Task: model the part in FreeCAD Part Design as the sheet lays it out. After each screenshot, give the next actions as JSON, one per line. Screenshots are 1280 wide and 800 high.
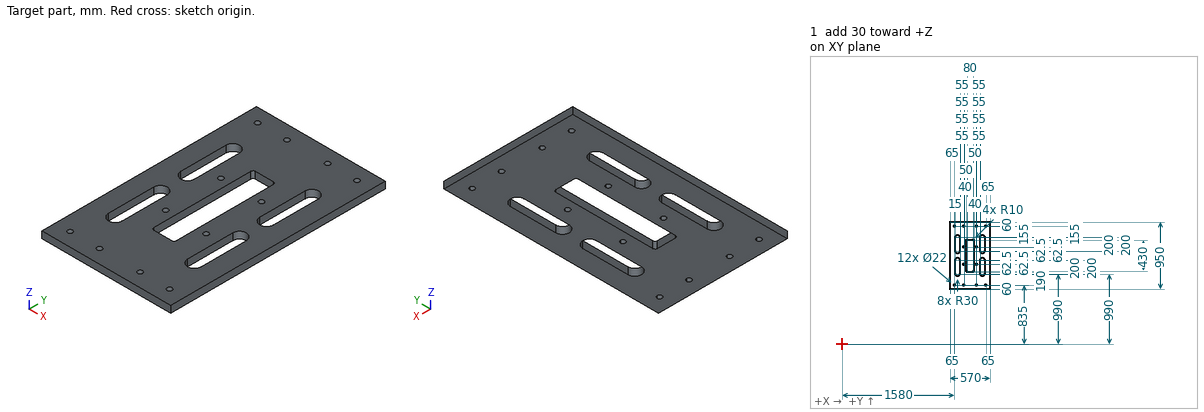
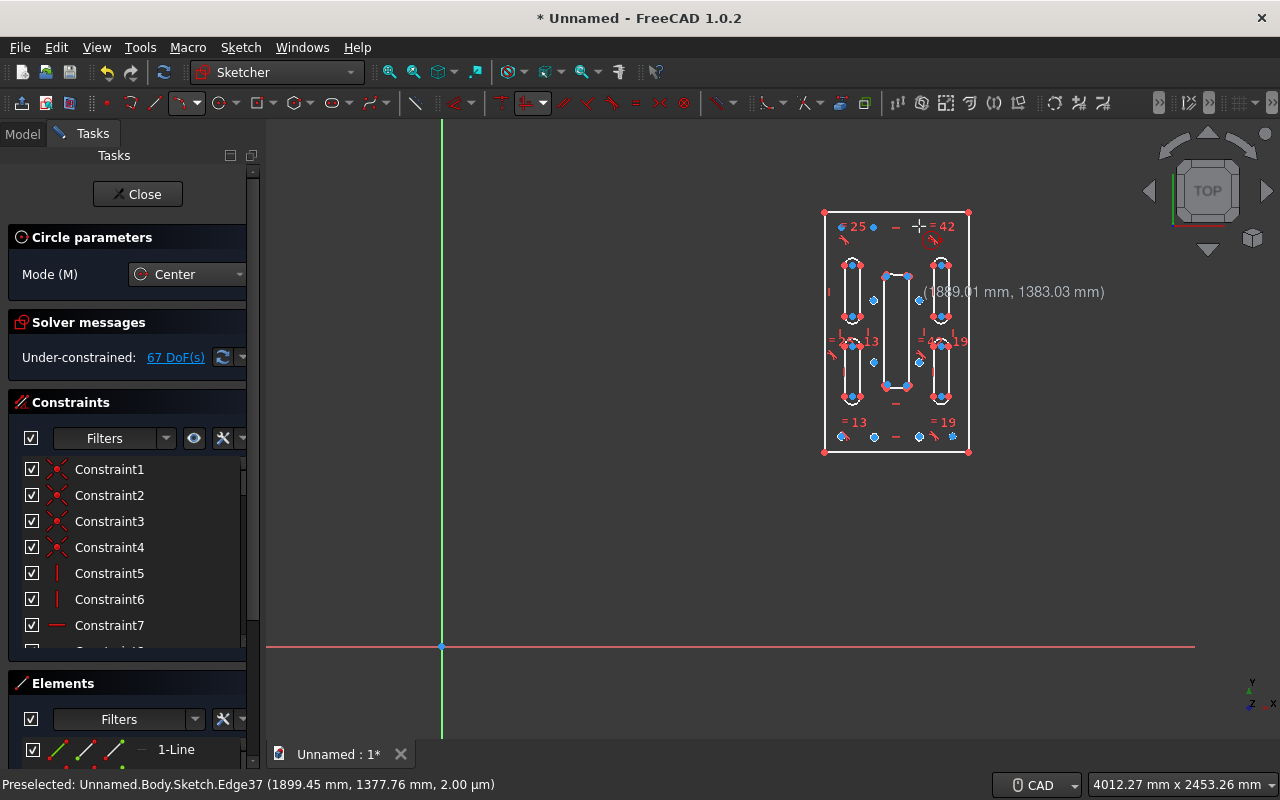
{"action": "left_click", "coordinate": [919, 226]}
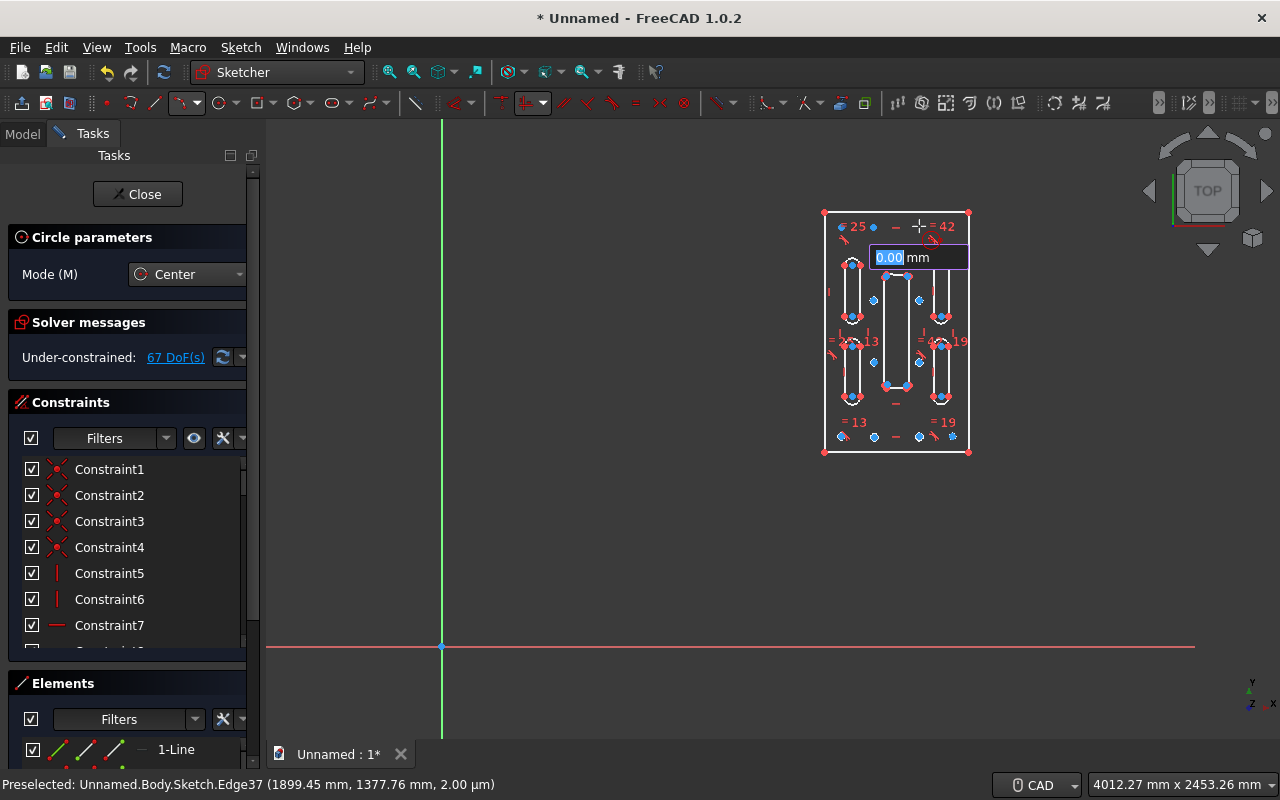
{"action": "scroll", "coordinate": [921, 228], "scroll_direction": "up", "scroll_amount": 9}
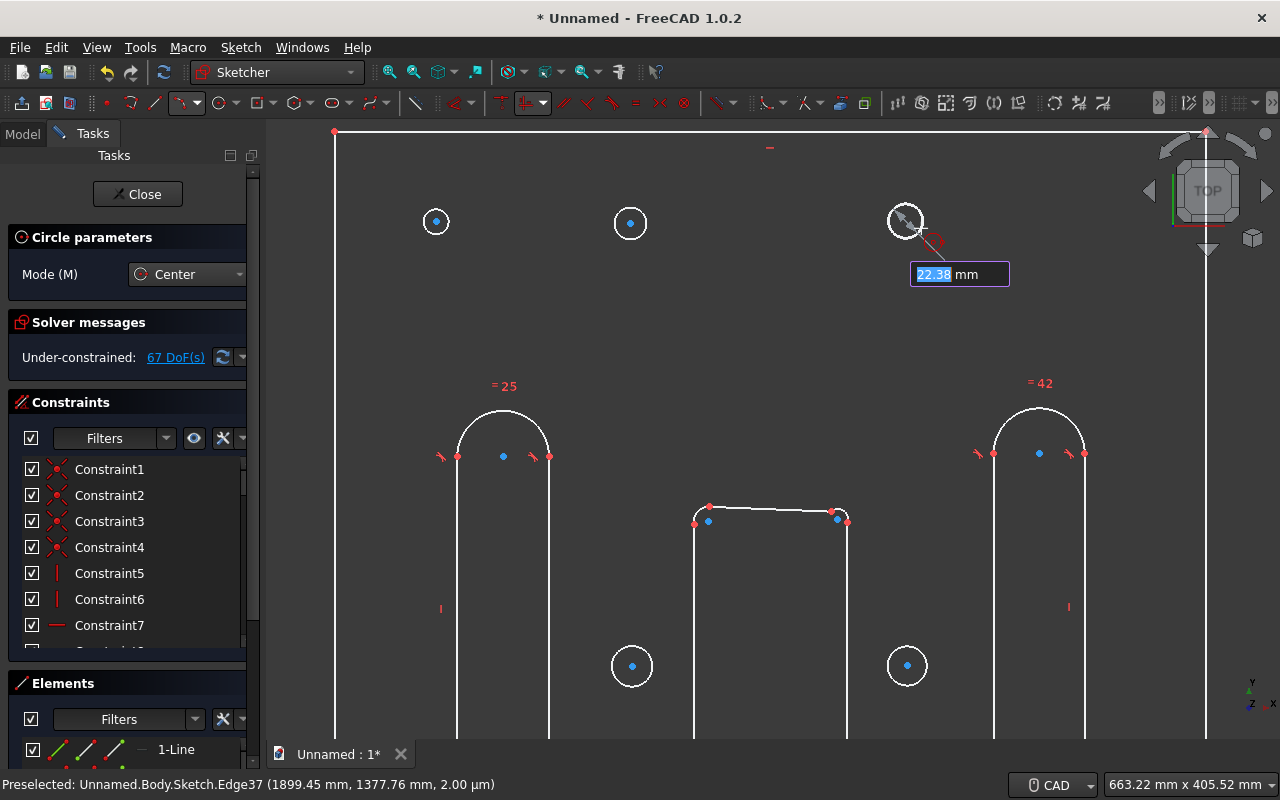
{"action": "left_click", "coordinate": [921, 227]}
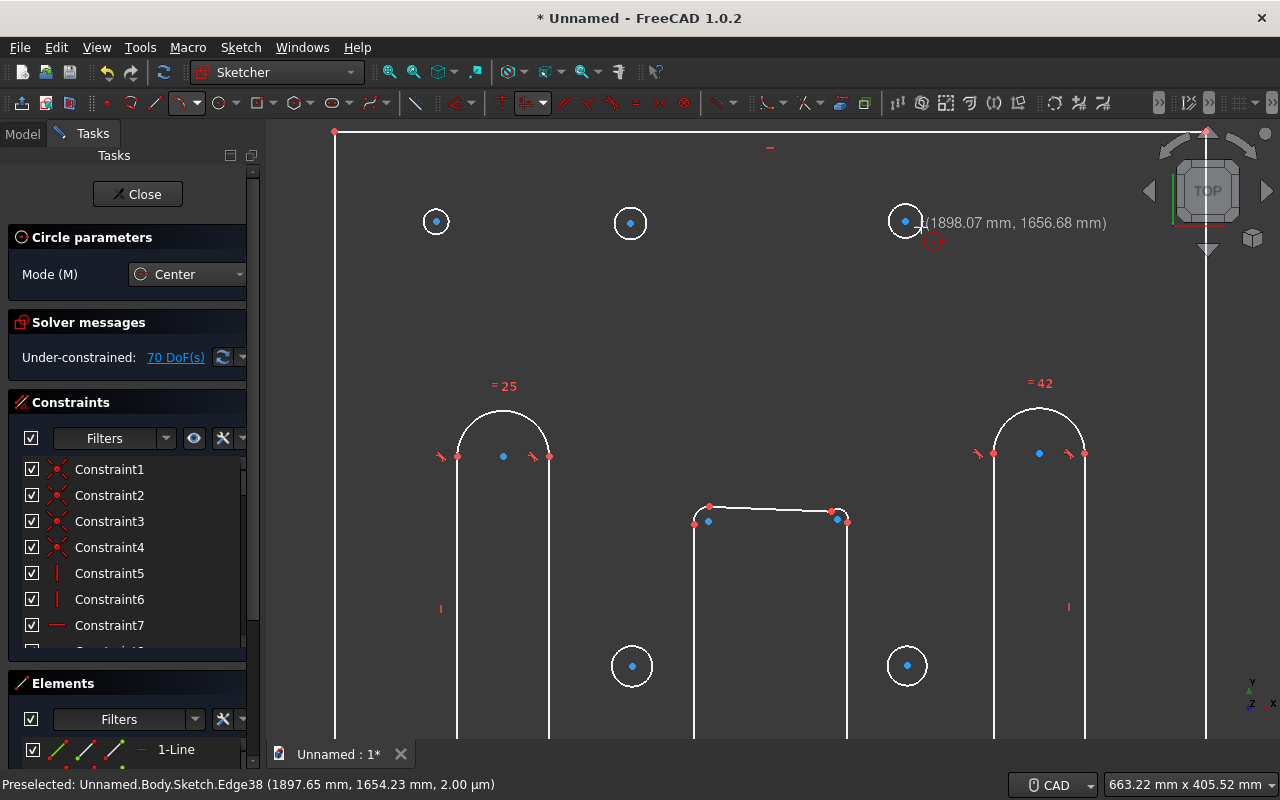
{"action": "scroll", "coordinate": [1107, 215], "scroll_direction": "up", "scroll_amount": 2}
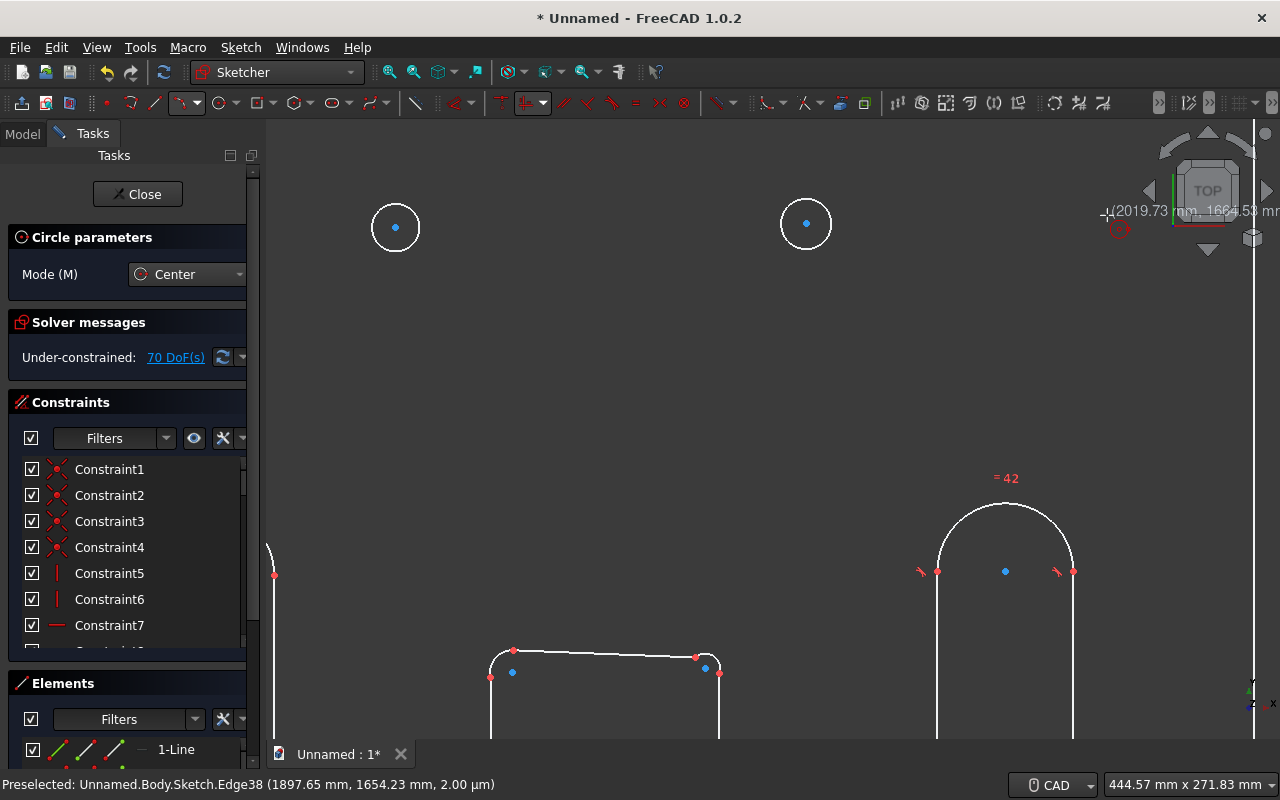
{"action": "scroll", "coordinate": [932, 228], "scroll_direction": "down", "scroll_amount": 11}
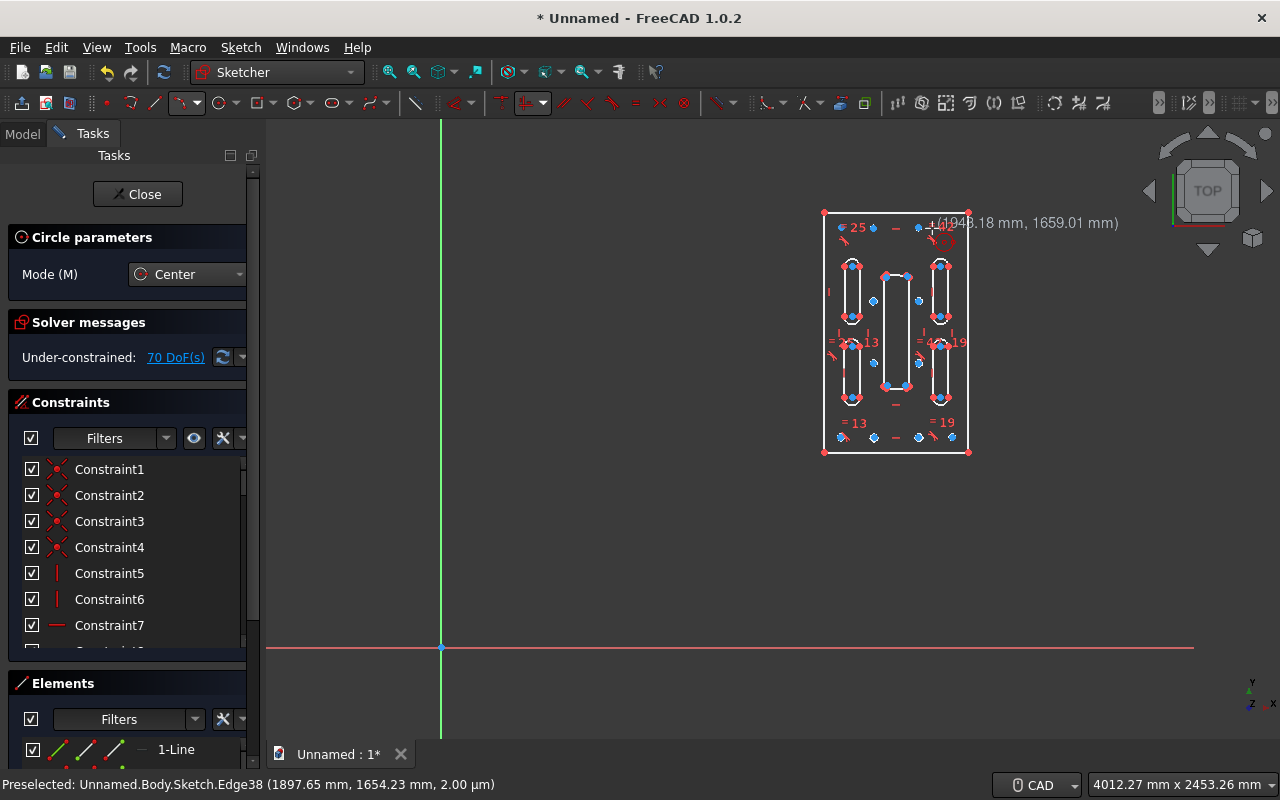
{"action": "left_click", "coordinate": [952, 227]}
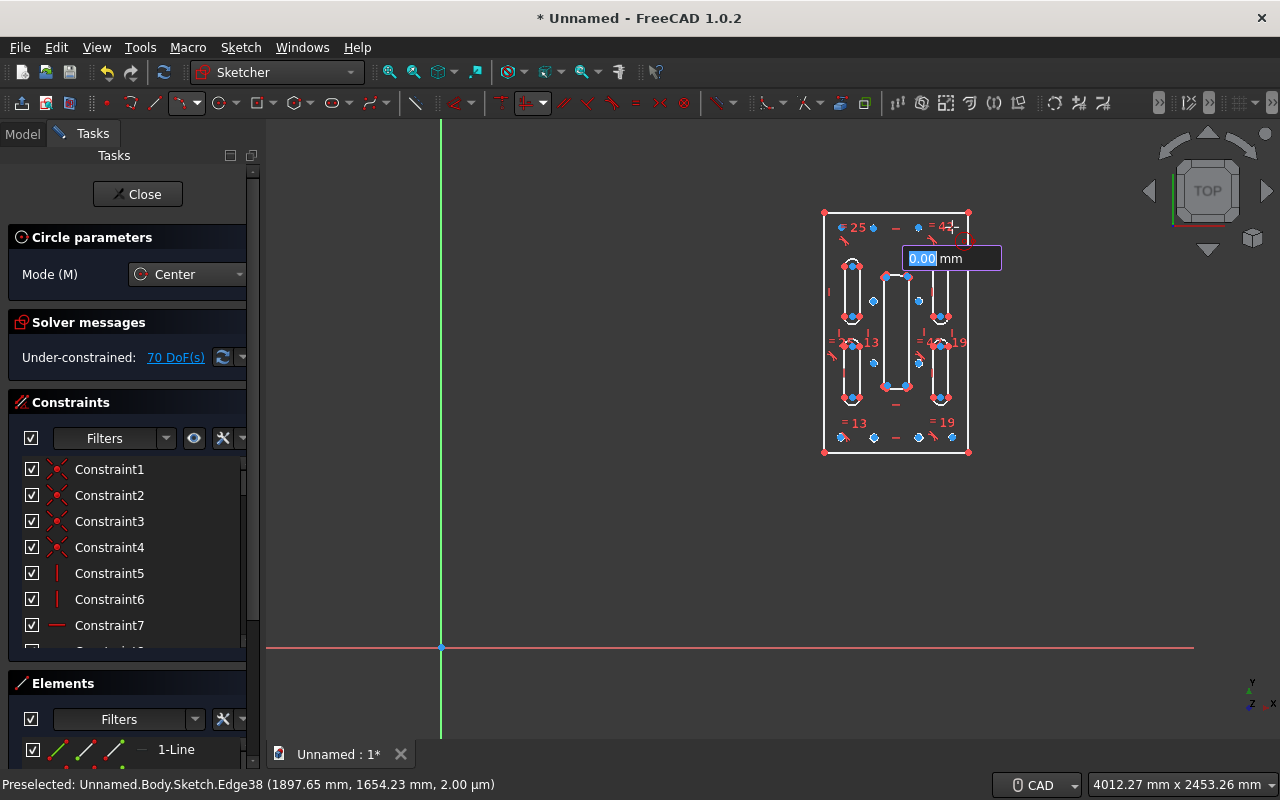
{"action": "scroll", "coordinate": [954, 229], "scroll_direction": "up", "scroll_amount": 9}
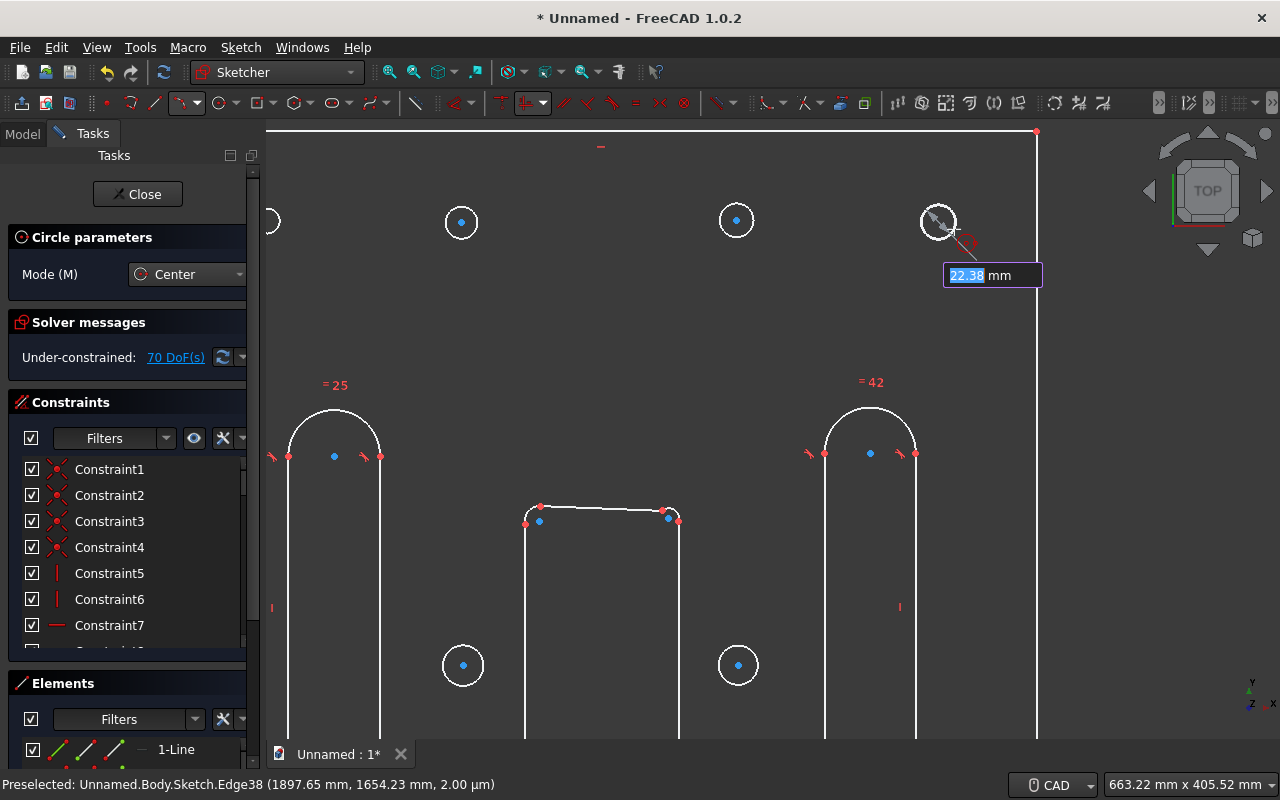
{"action": "left_click", "coordinate": [950, 226]}
{"action": "key", "text": "Escape"}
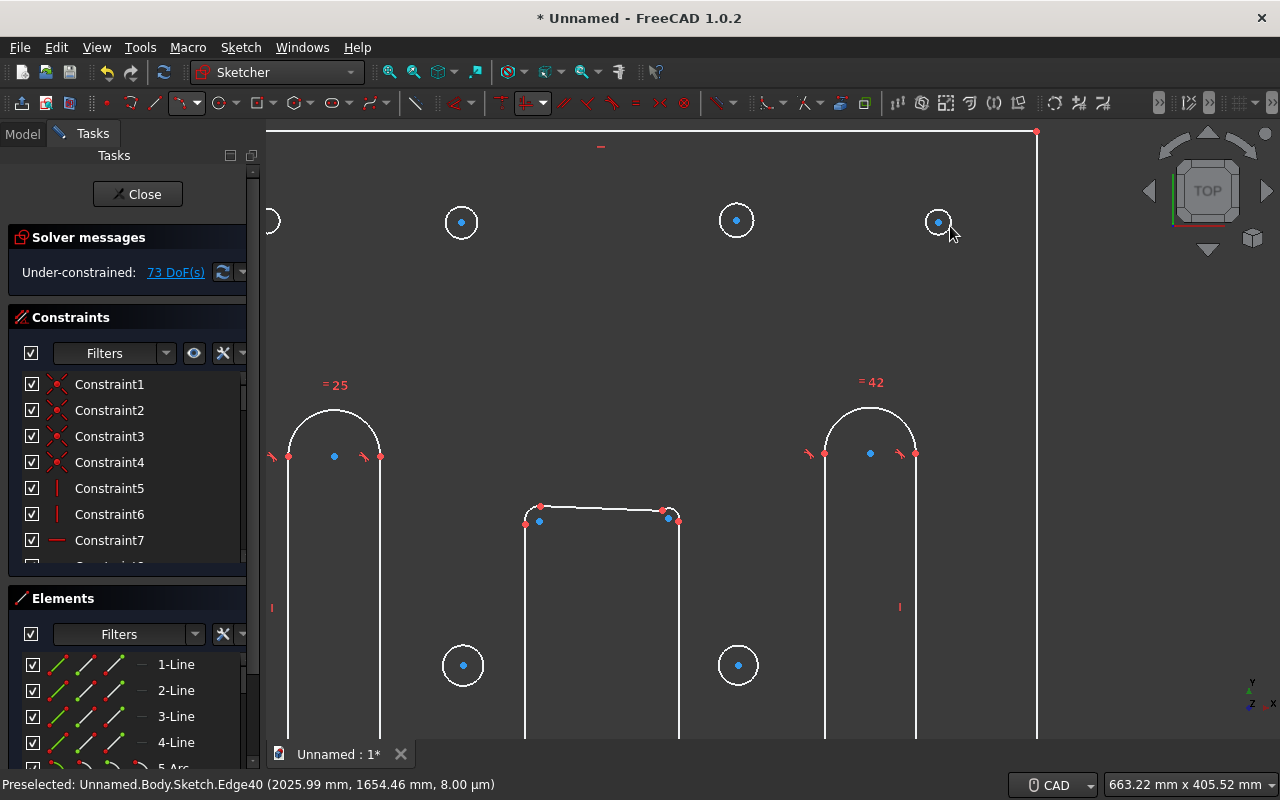
{"action": "scroll", "coordinate": [954, 228], "scroll_direction": "down", "scroll_amount": 9}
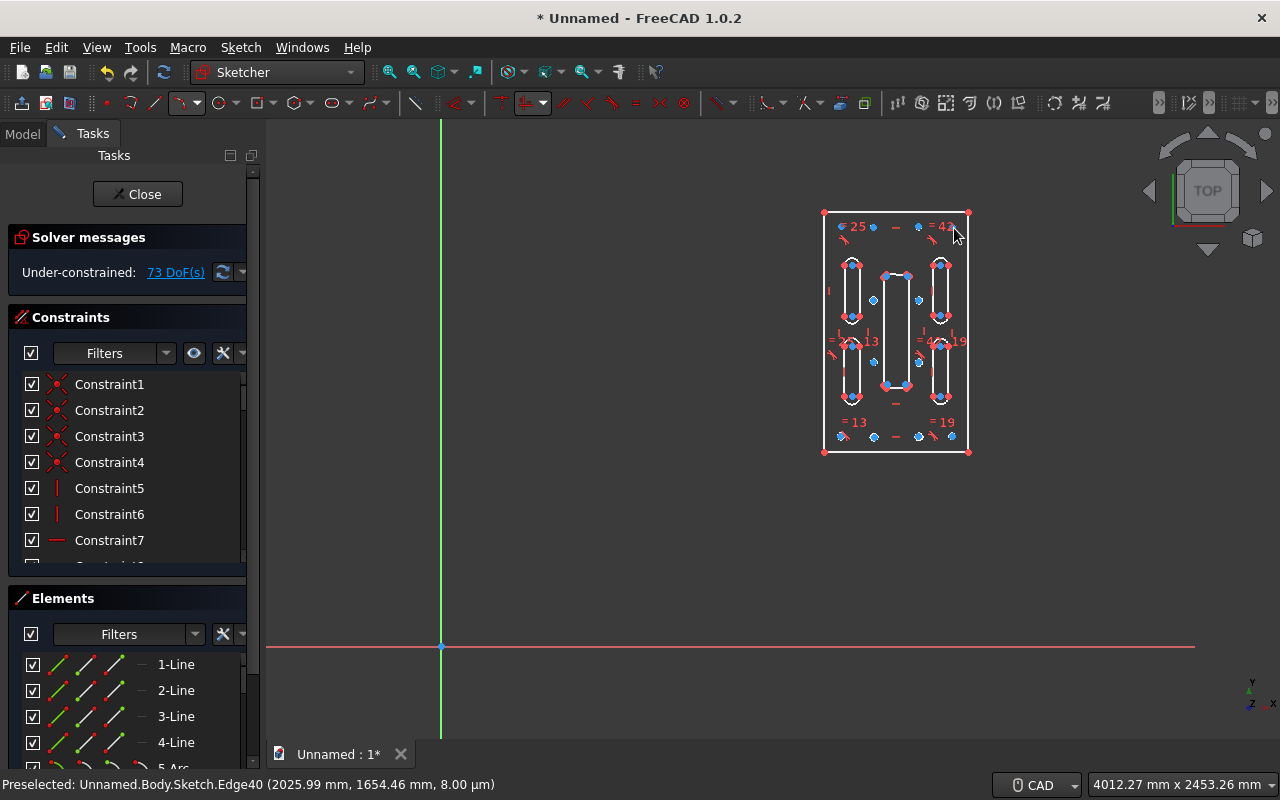
{"action": "scroll", "coordinate": [900, 388], "scroll_direction": "up", "scroll_amount": 5}